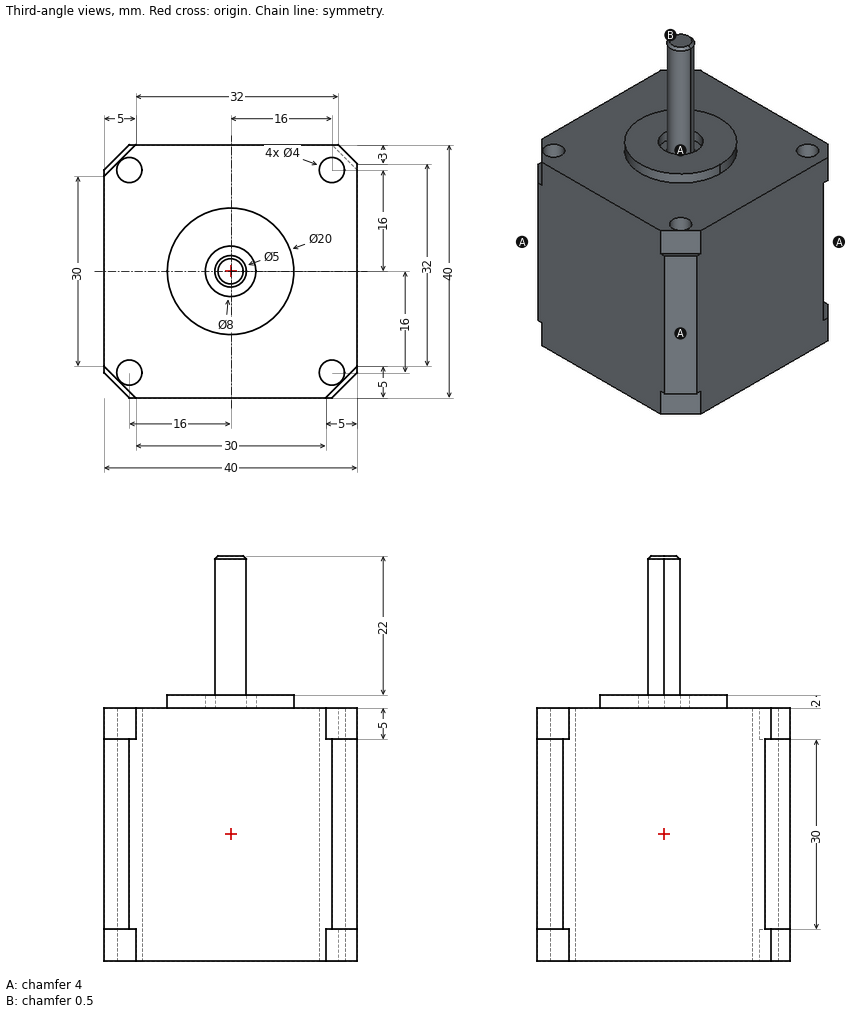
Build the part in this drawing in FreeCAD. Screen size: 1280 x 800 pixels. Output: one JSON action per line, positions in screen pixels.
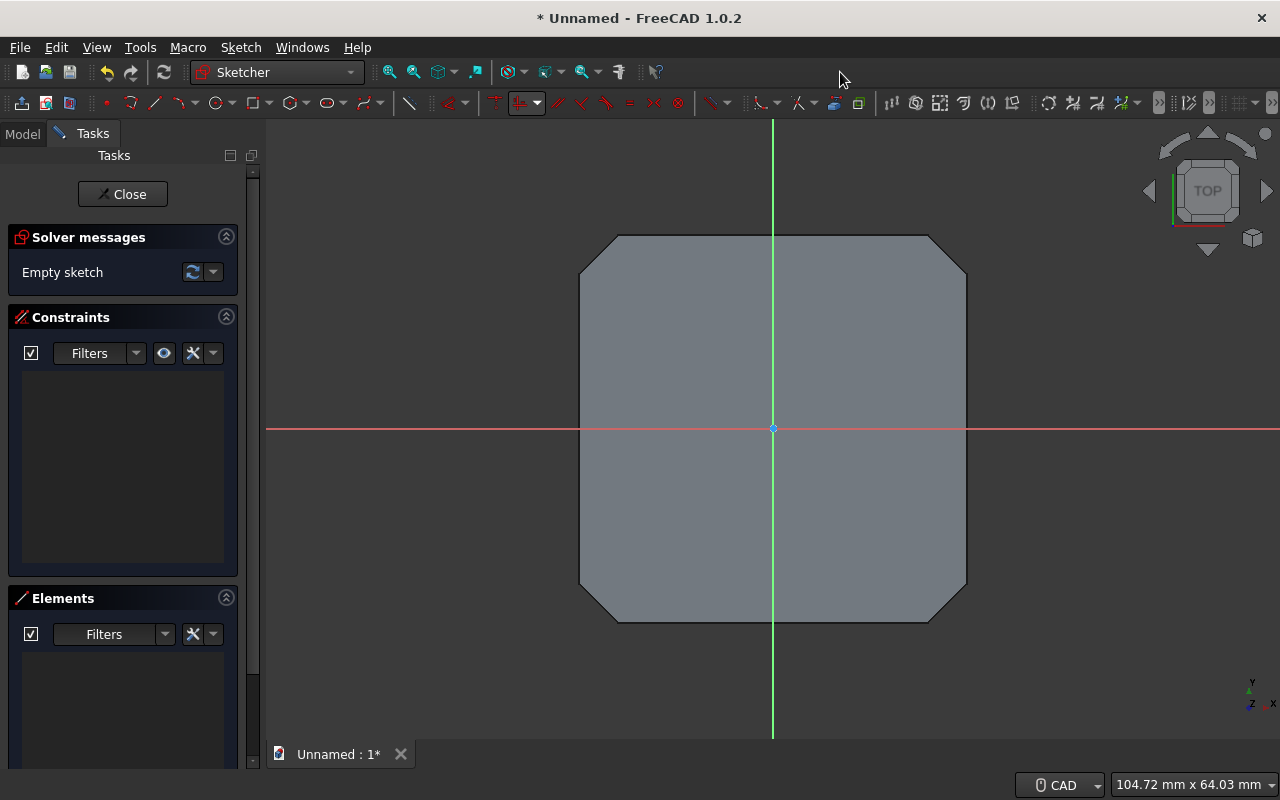
{"action": "left_click", "coordinate": [132, 104]}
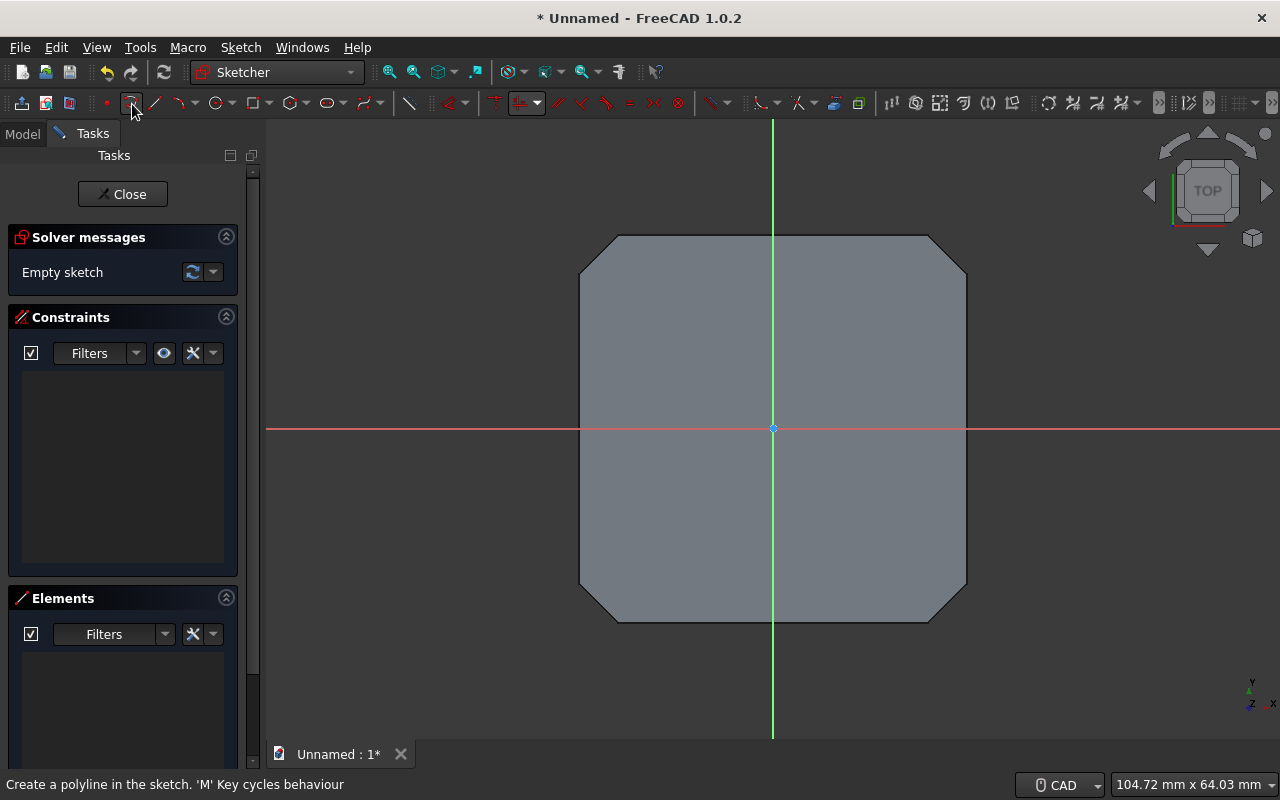
{"action": "left_click", "coordinate": [628, 623]}
{"action": "left_click", "coordinate": [918, 623]}
{"action": "left_click", "coordinate": [967, 574]}
{"action": "left_click", "coordinate": [967, 264]}
{"action": "left_click", "coordinate": [938, 235]}
{"action": "left_click", "coordinate": [628, 235]}
{"action": "left_click", "coordinate": [579, 284]}
{"action": "left_click", "coordinate": [579, 574]}
{"action": "left_click", "coordinate": [628, 624]}
{"action": "key", "text": "Escape"}
{"action": "key", "text": "Escape"}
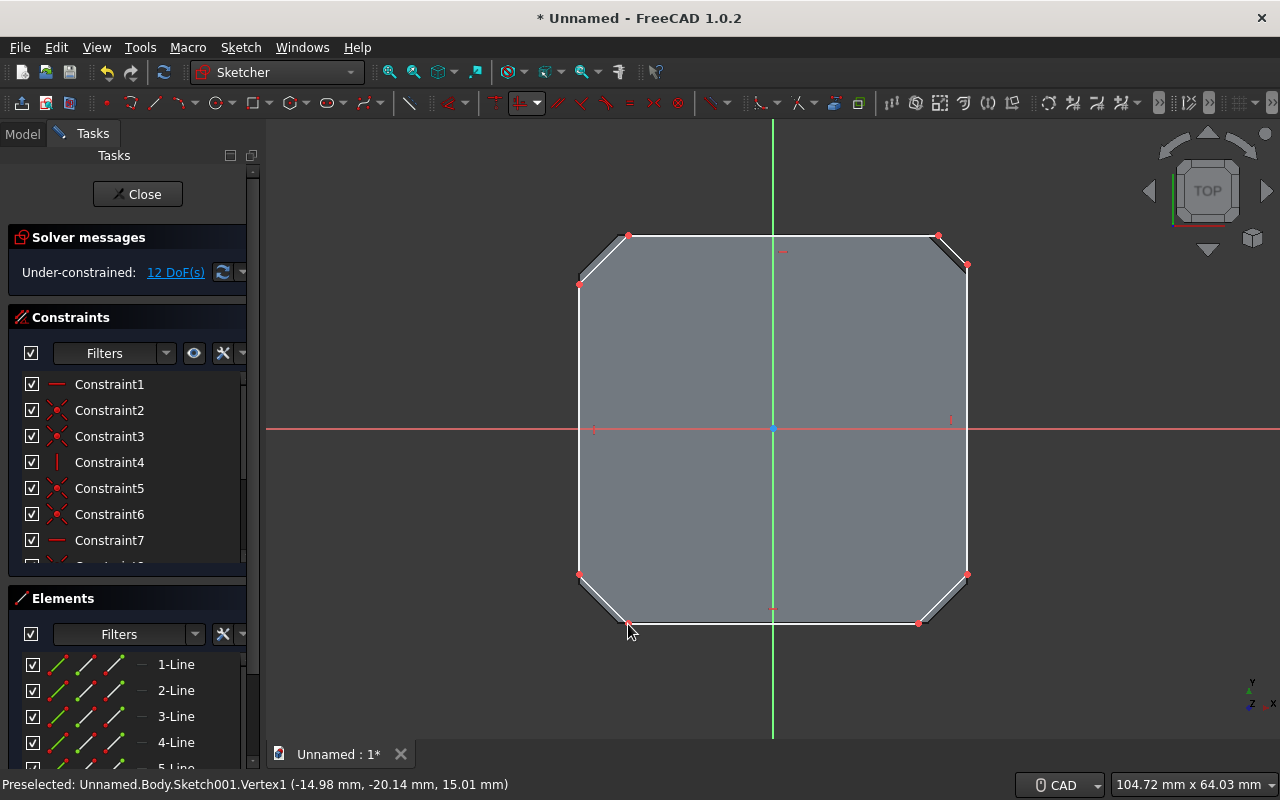
{"action": "left_click", "coordinate": [628, 624]}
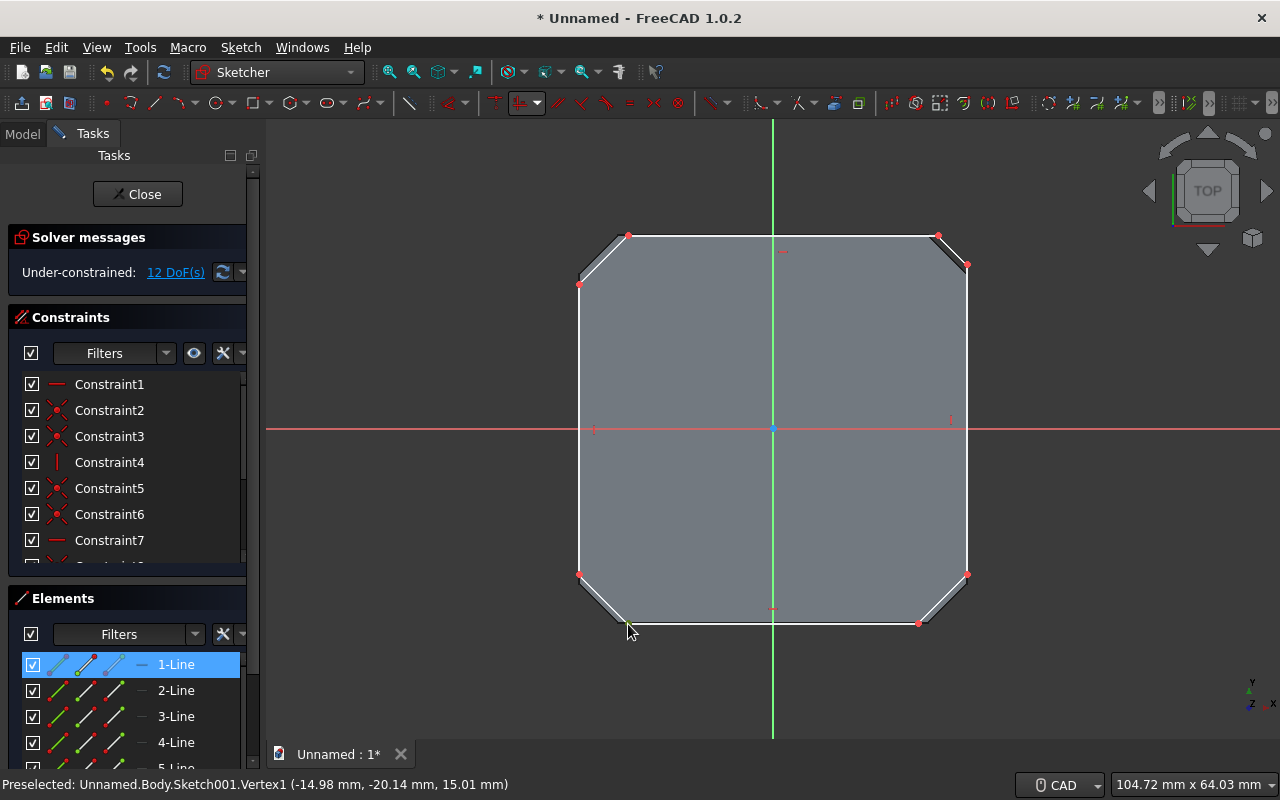
{"action": "left_click", "coordinate": [628, 236]}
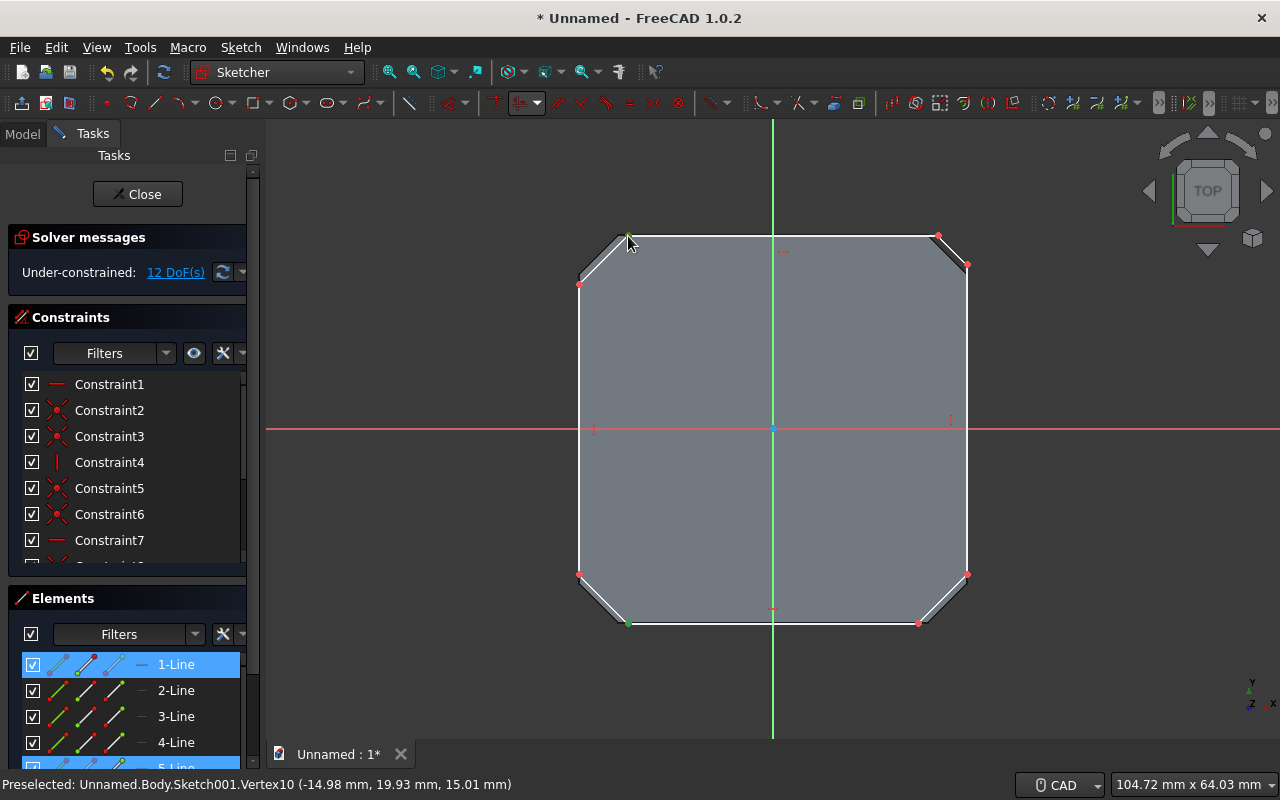
{"action": "left_click", "coordinate": [353, 429]}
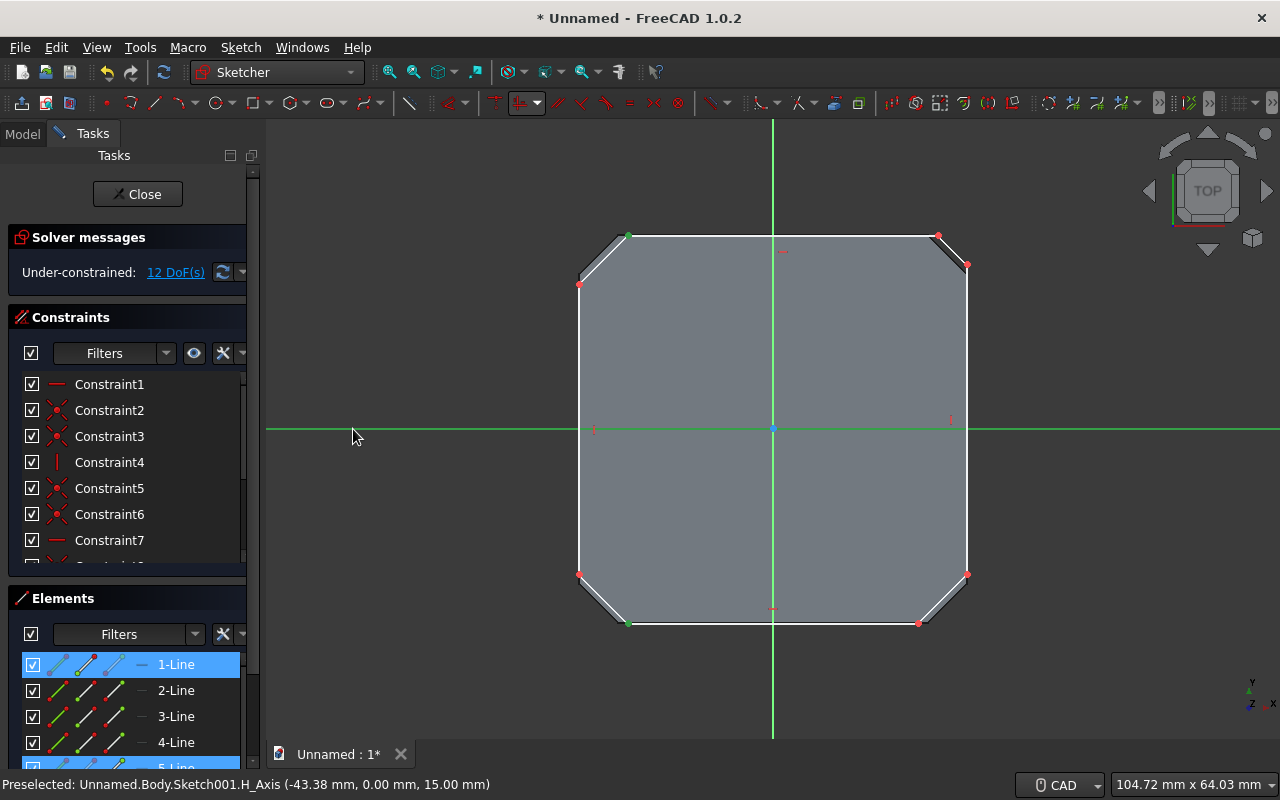
{"action": "left_click", "coordinate": [654, 104]}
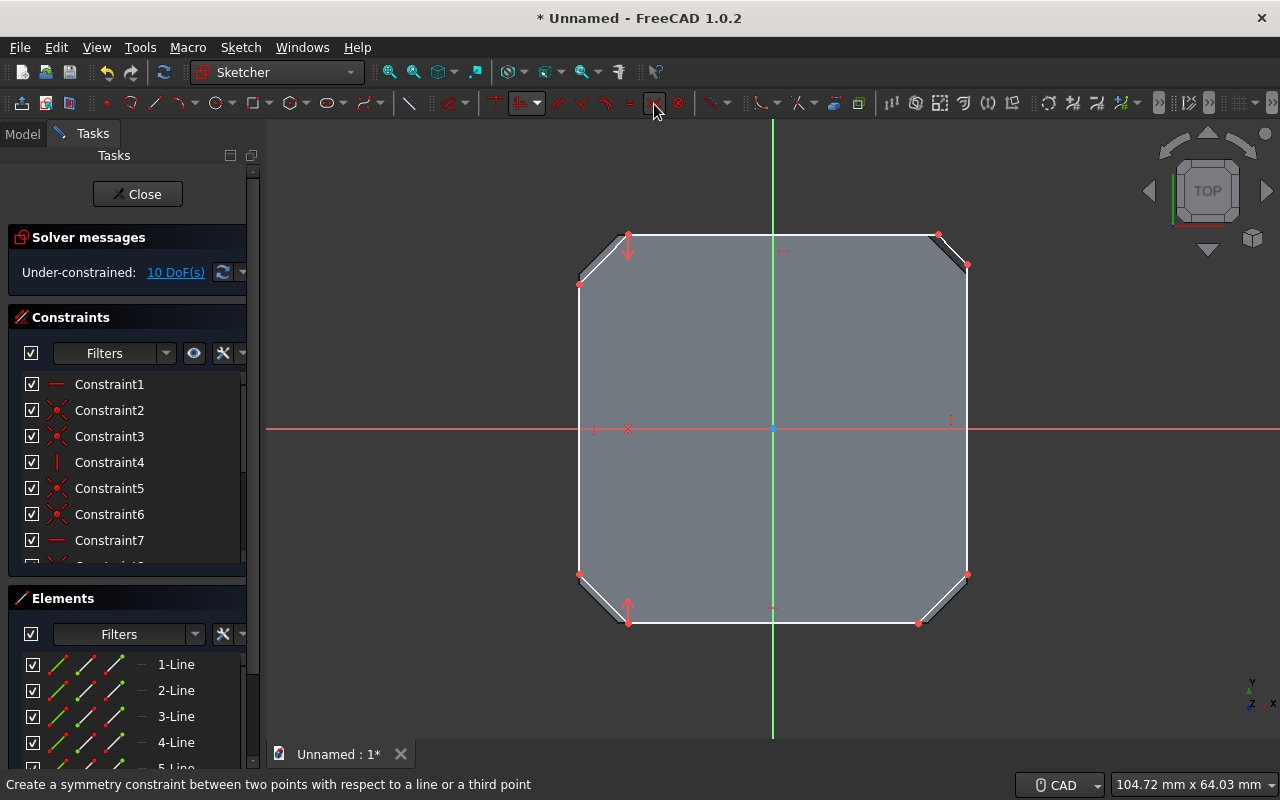
{"action": "left_click", "coordinate": [967, 575]}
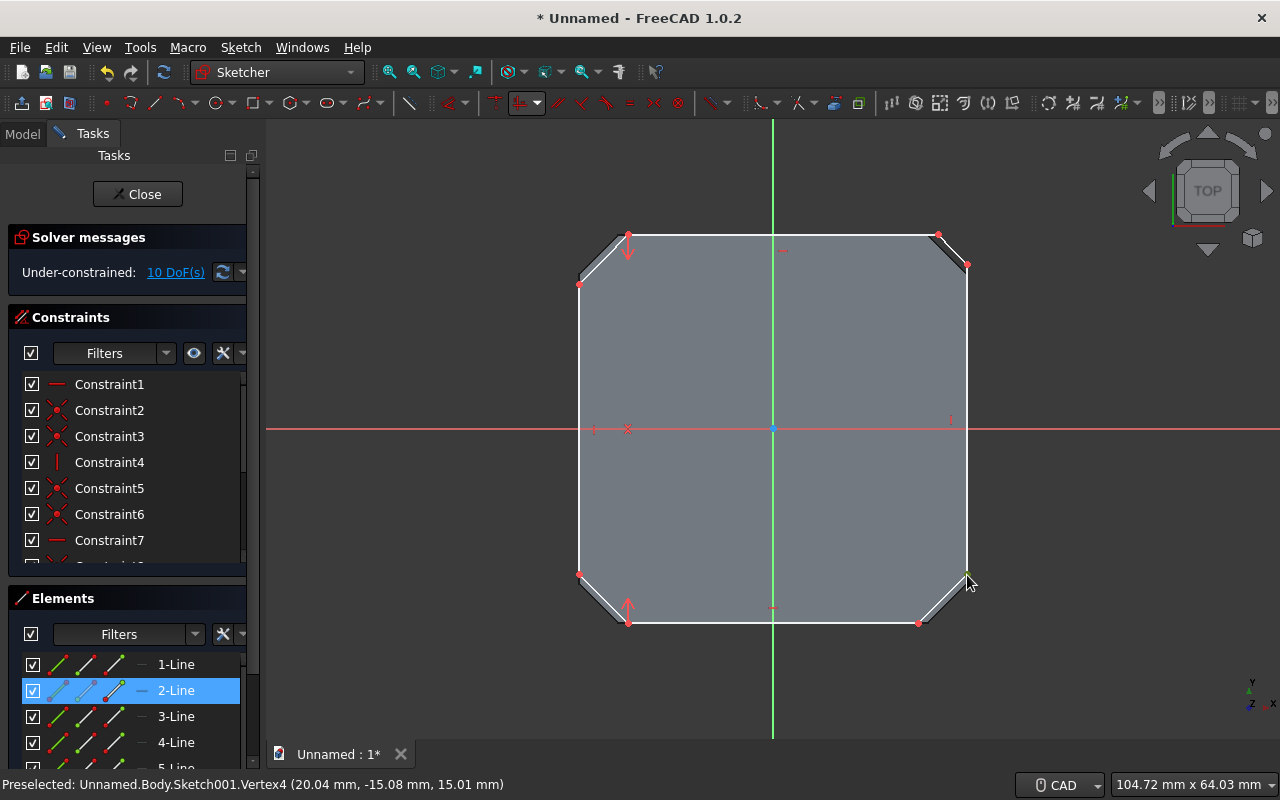
{"action": "left_click", "coordinate": [579, 575]}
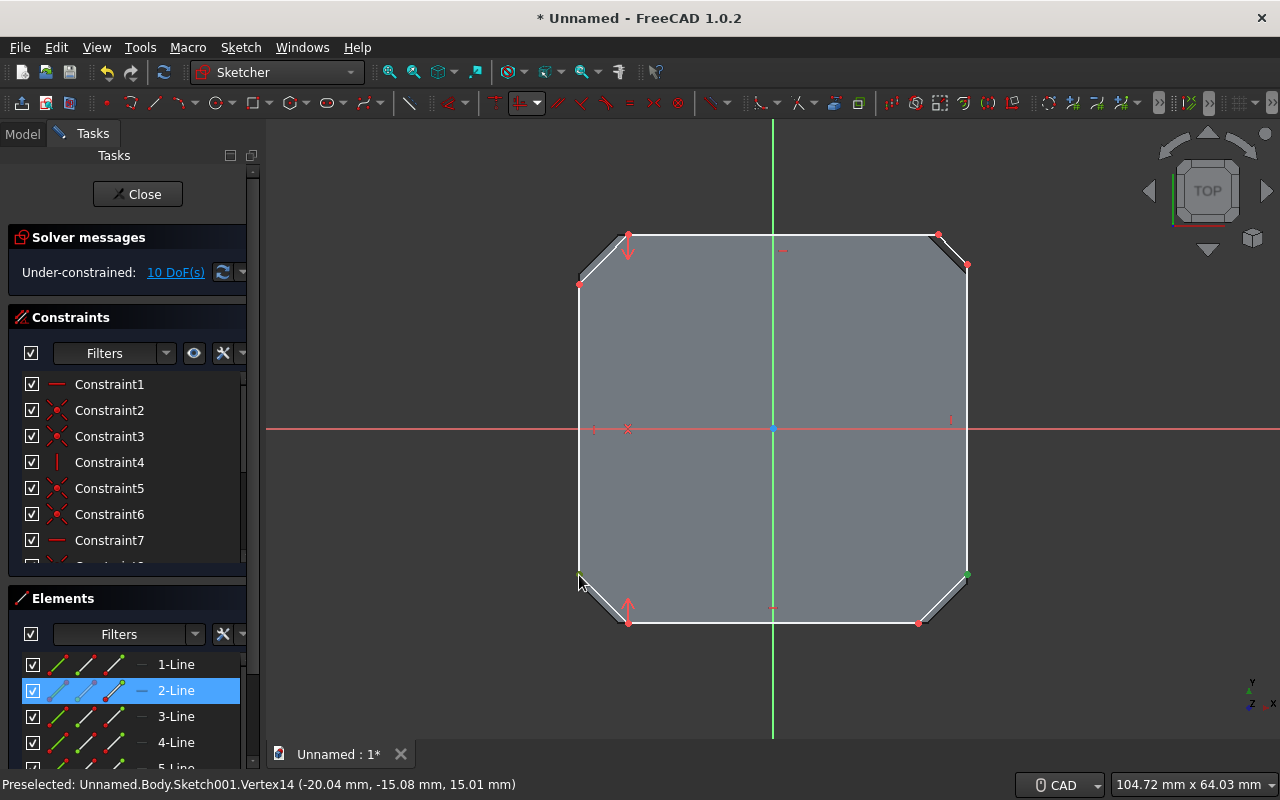
{"action": "left_click", "coordinate": [773, 671]}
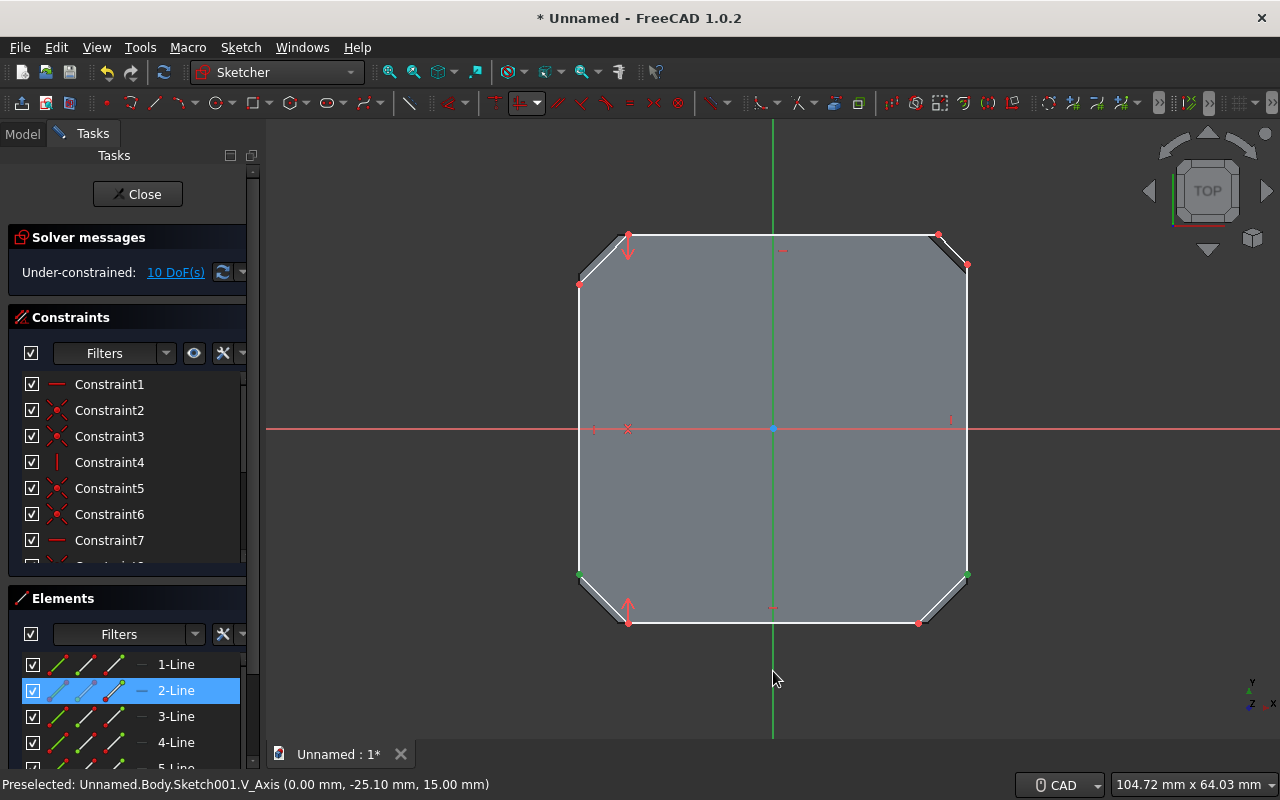
{"action": "left_click", "coordinate": [654, 104]}